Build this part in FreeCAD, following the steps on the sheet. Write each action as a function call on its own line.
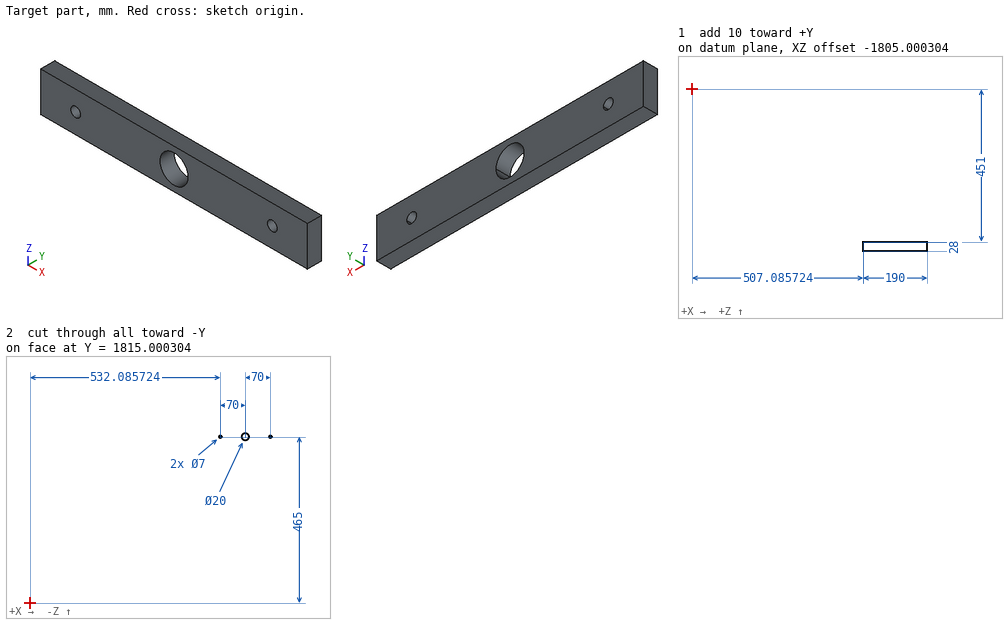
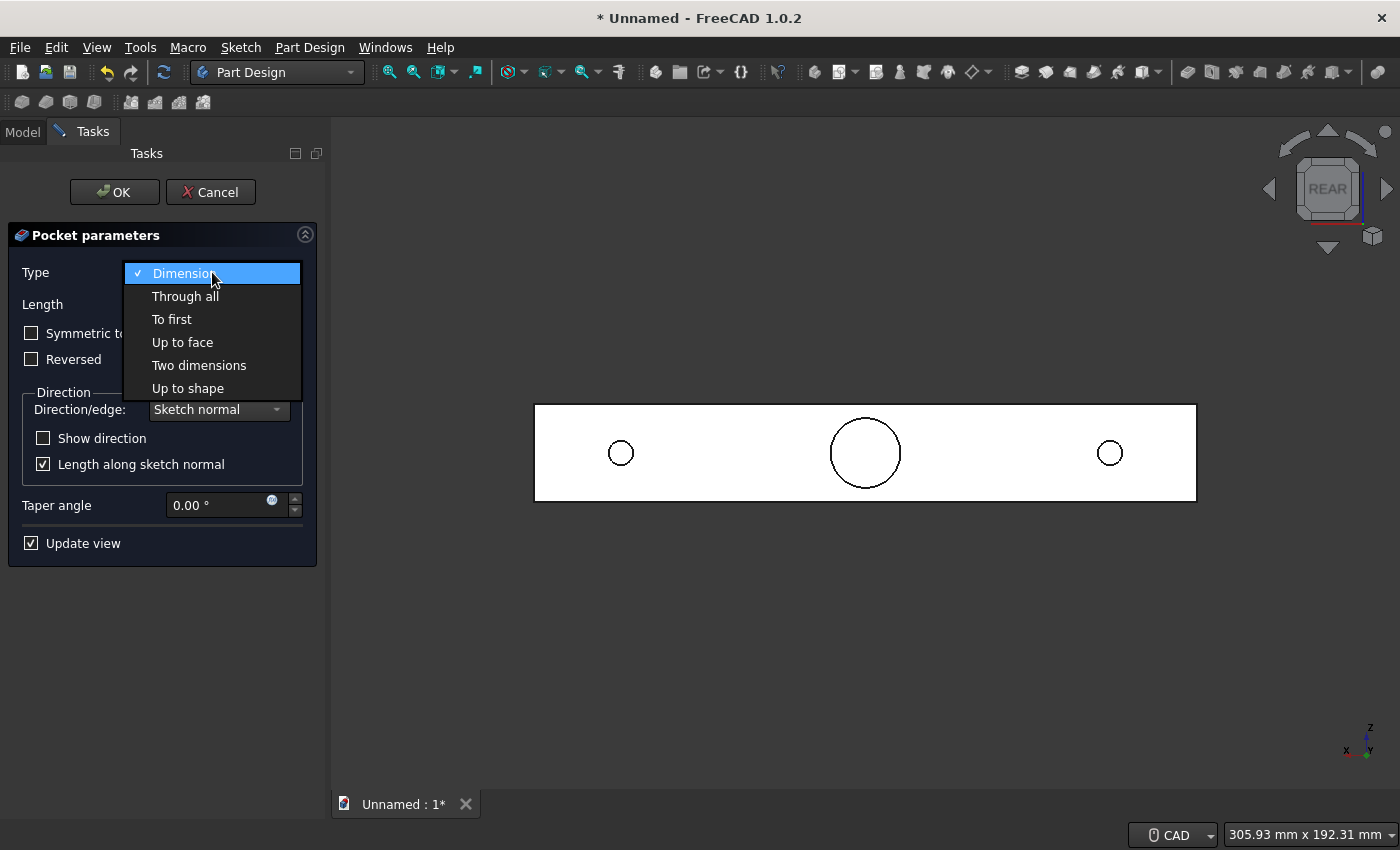
click(212, 296)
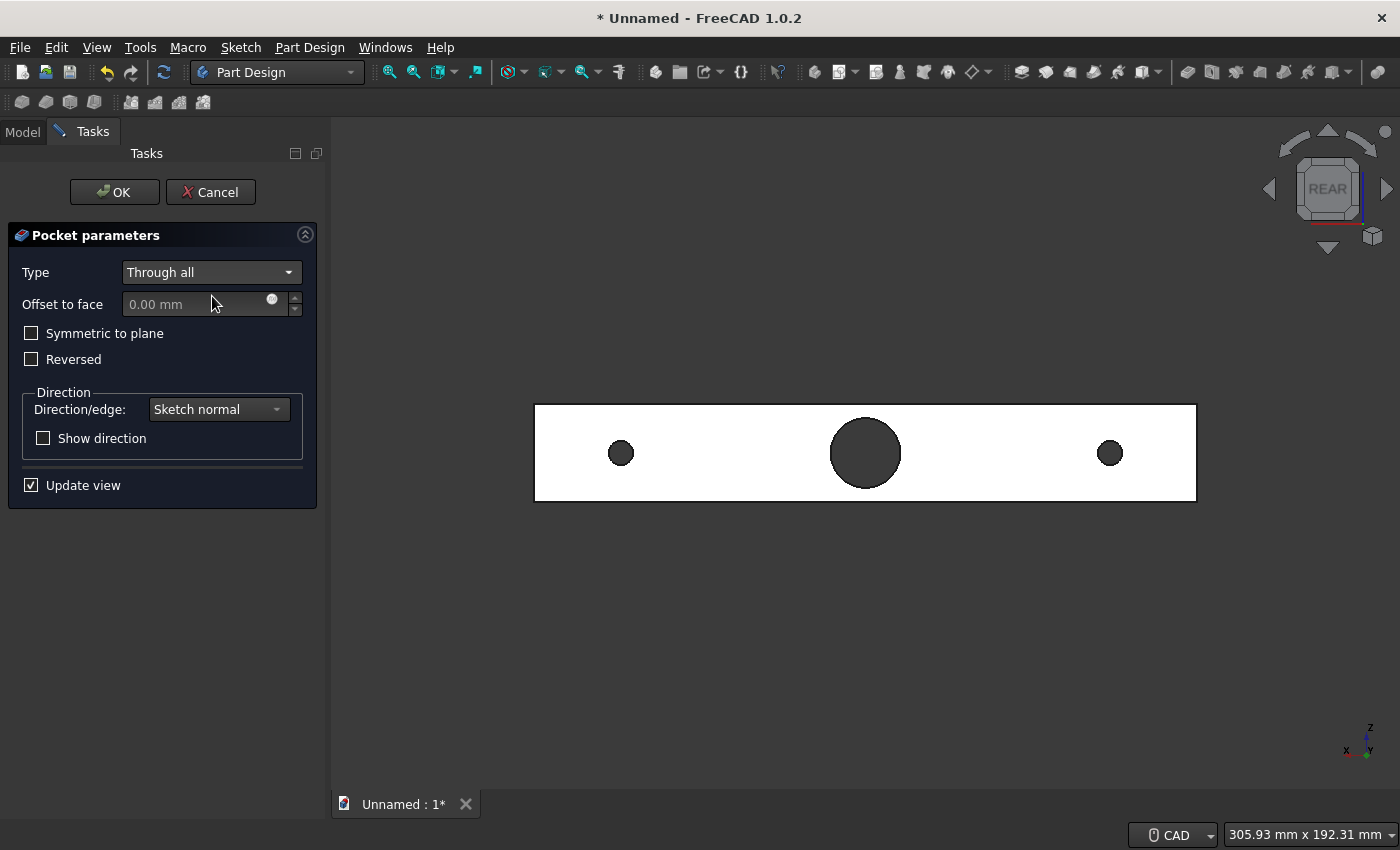
click(115, 192)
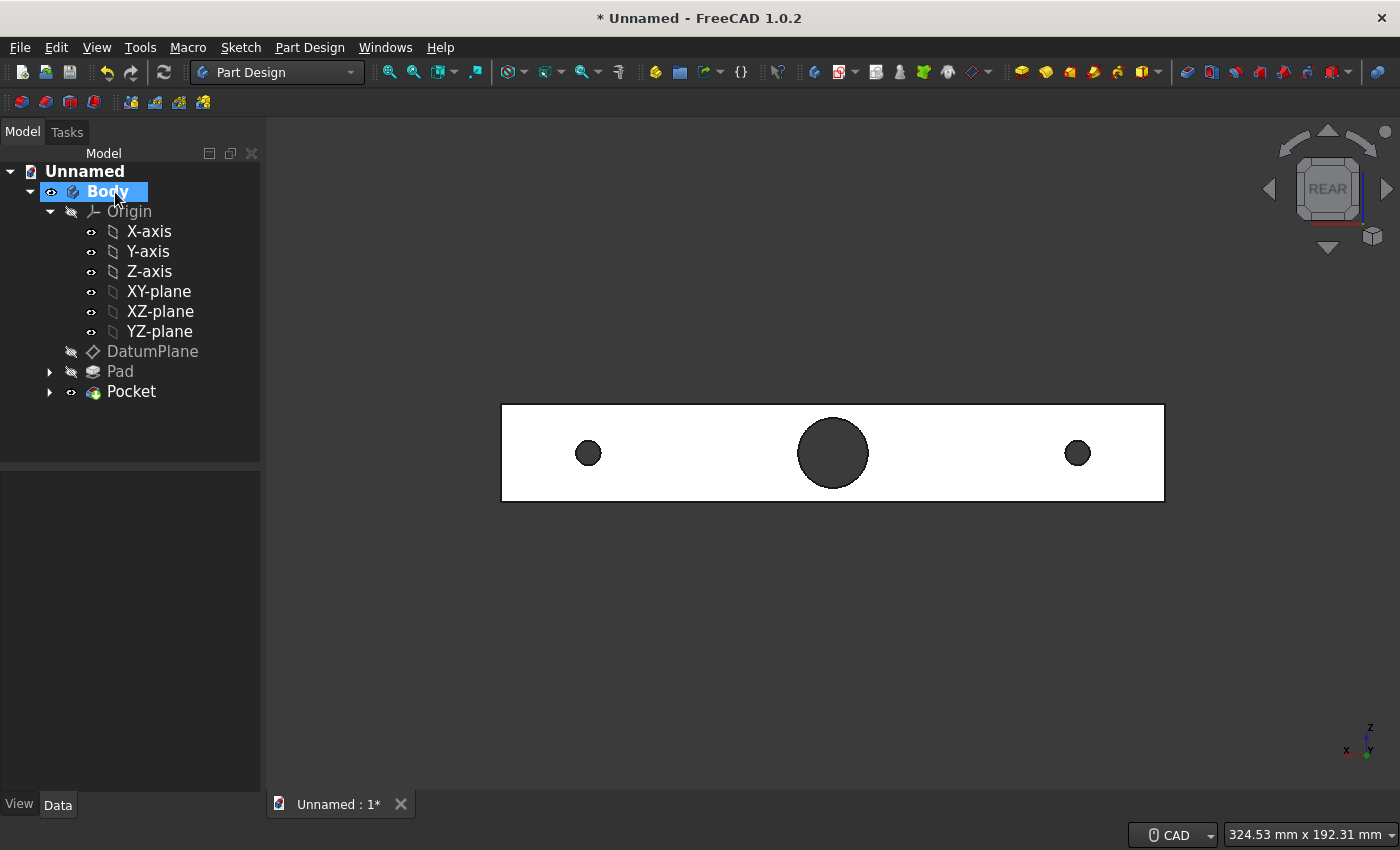
key(0)